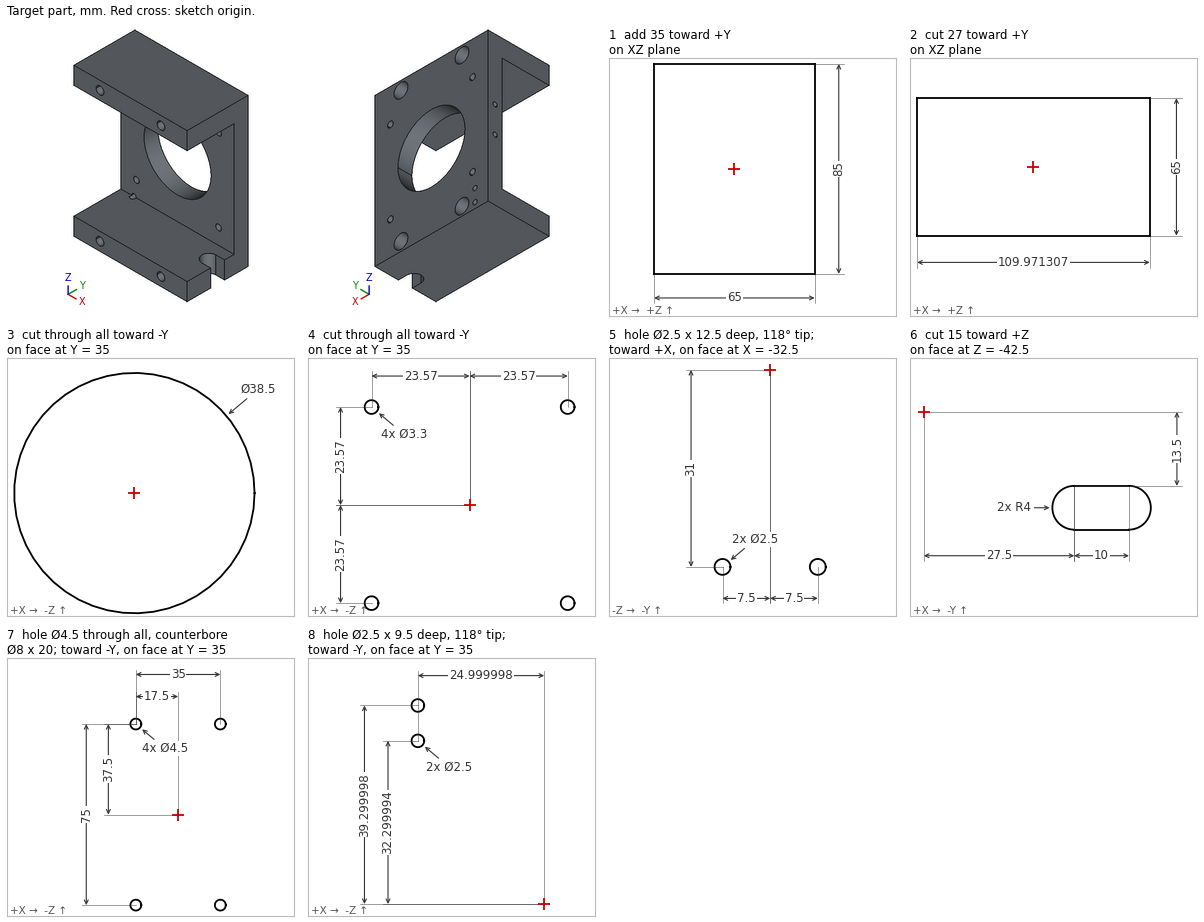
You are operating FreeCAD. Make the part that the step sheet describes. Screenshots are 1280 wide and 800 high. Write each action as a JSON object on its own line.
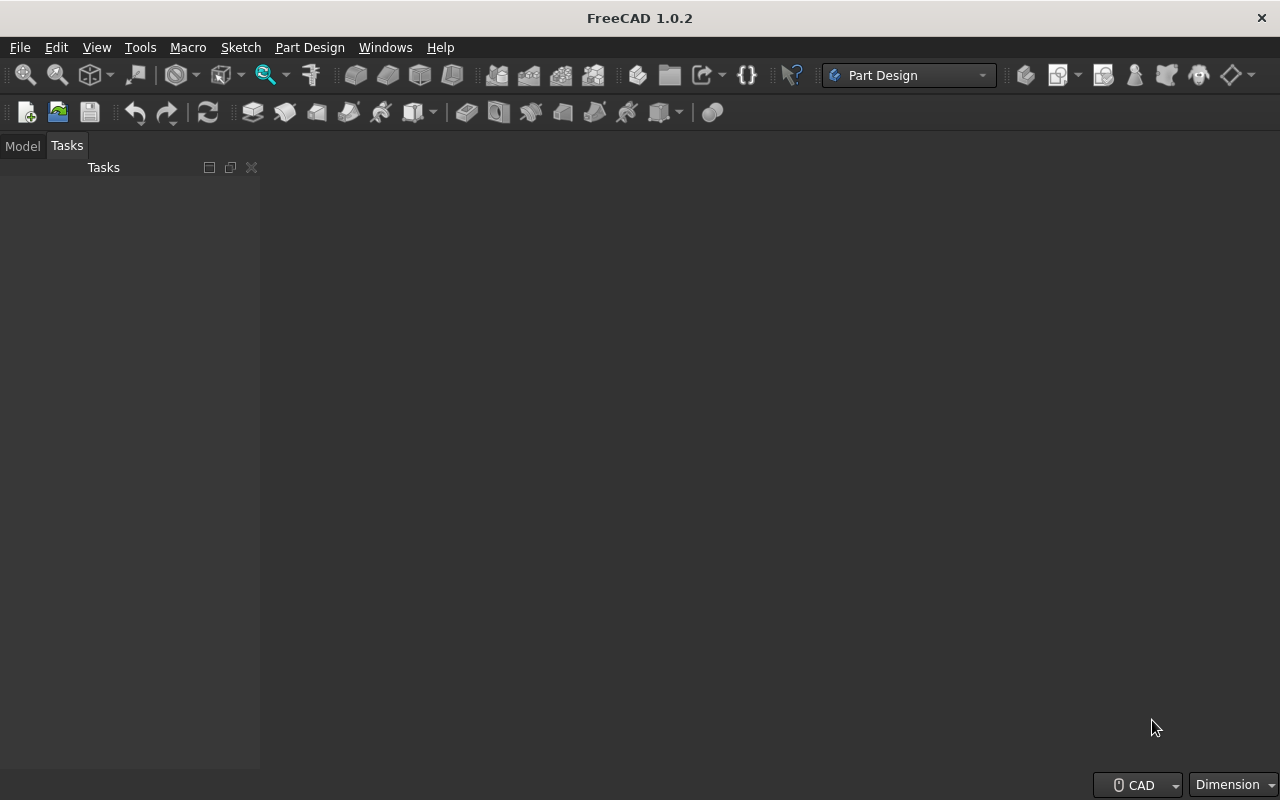
{"action": "left_click", "coordinate": [26, 112]}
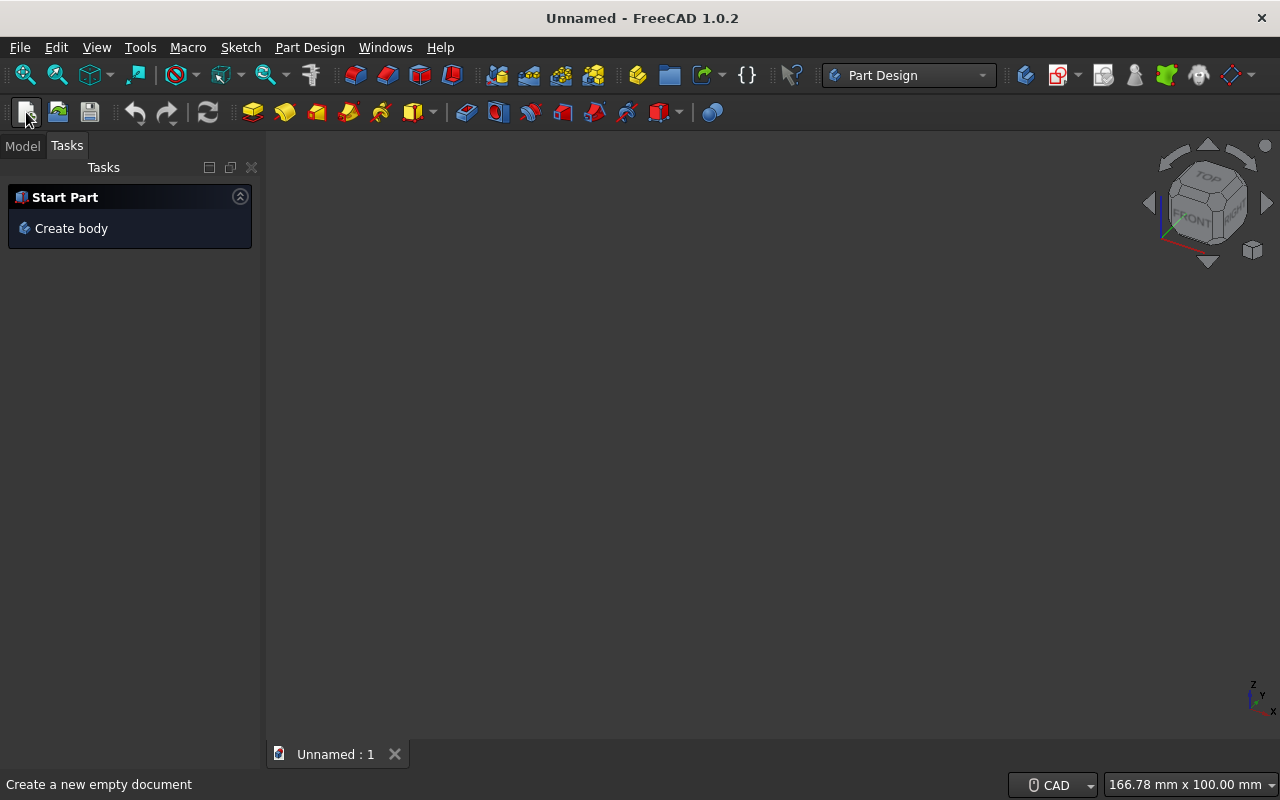
{"action": "left_click", "coordinate": [1058, 76]}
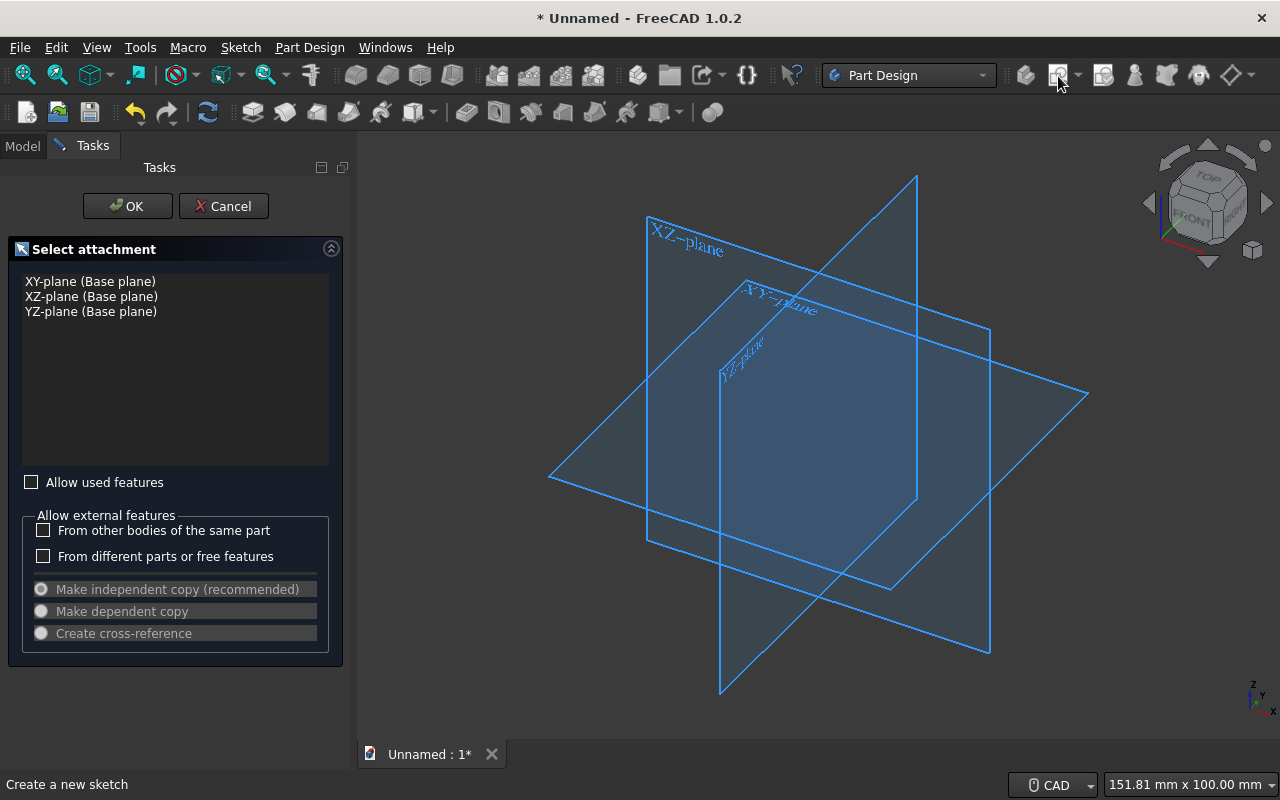
{"action": "left_click", "coordinate": [82, 296]}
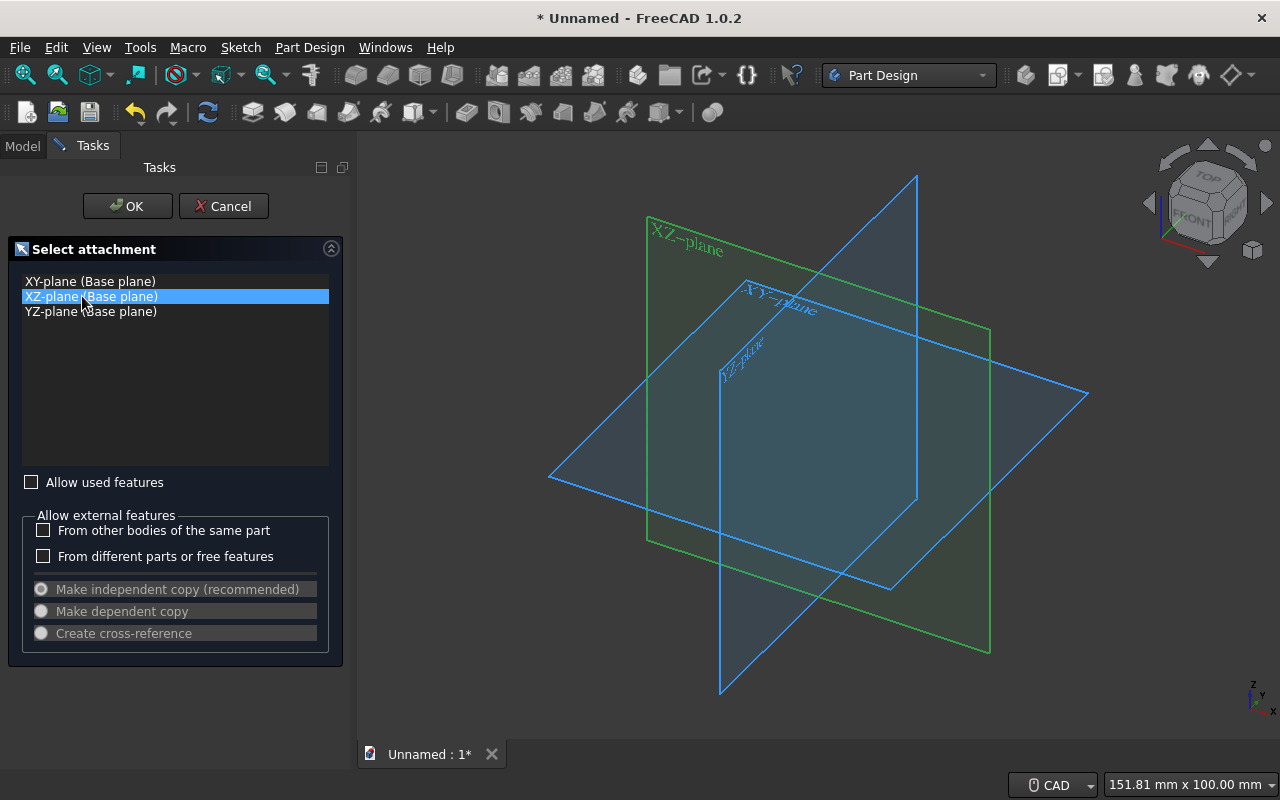
{"action": "left_click", "coordinate": [128, 206]}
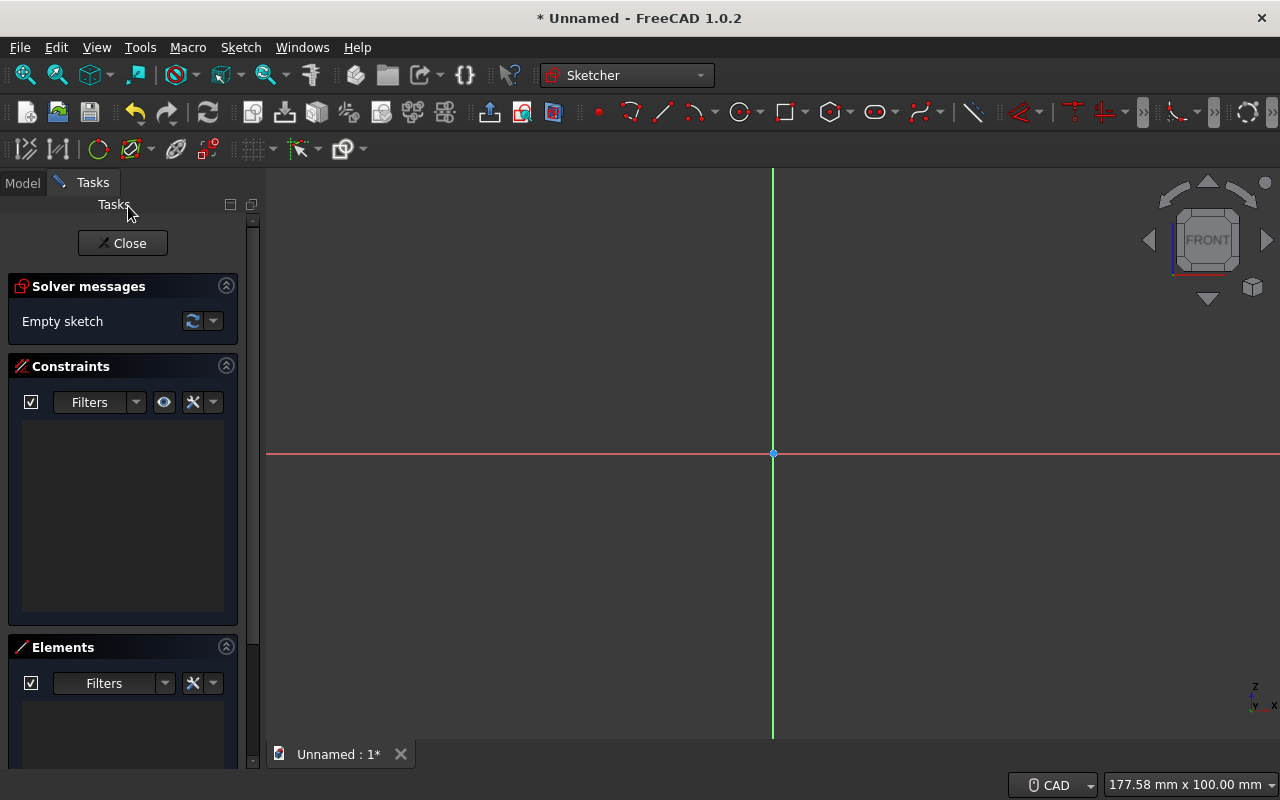
{"action": "scroll", "coordinate": [395, 453], "scroll_direction": "down", "scroll_amount": 1}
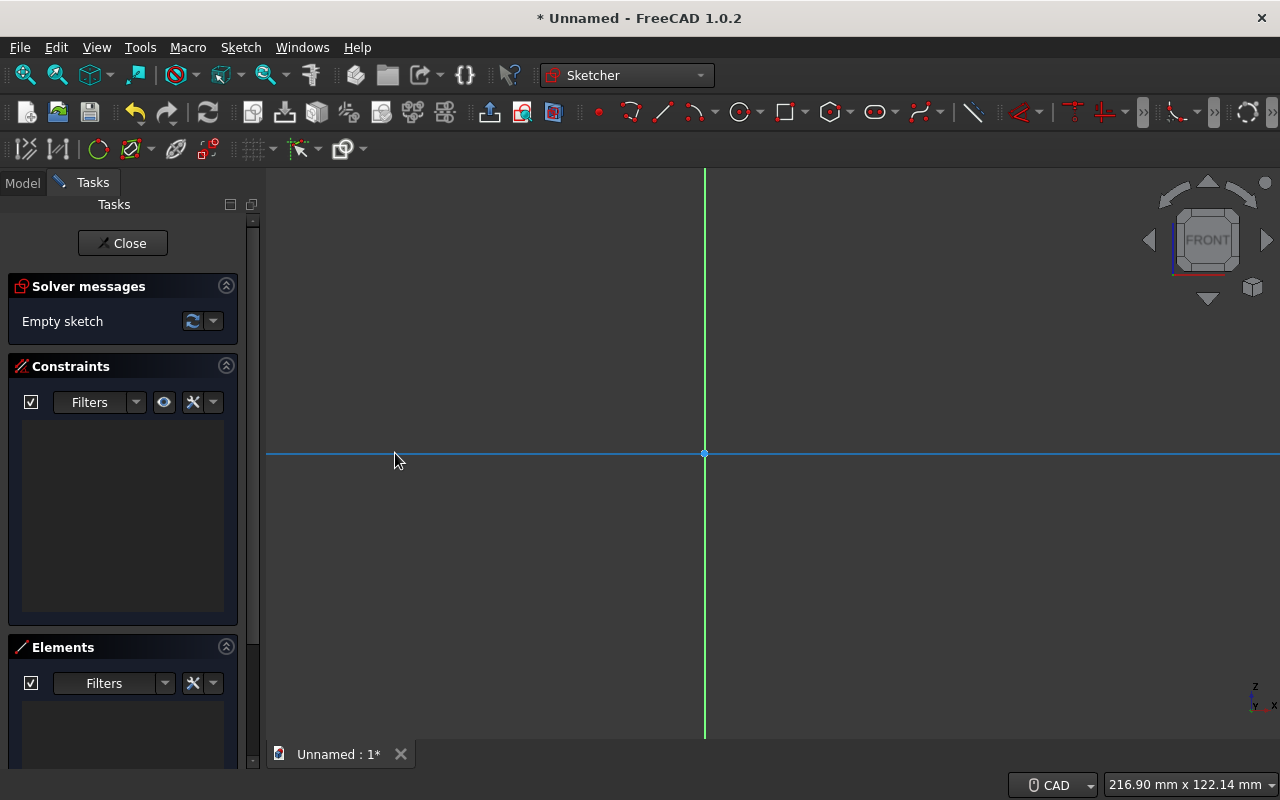
{"action": "left_click", "coordinate": [808, 112]}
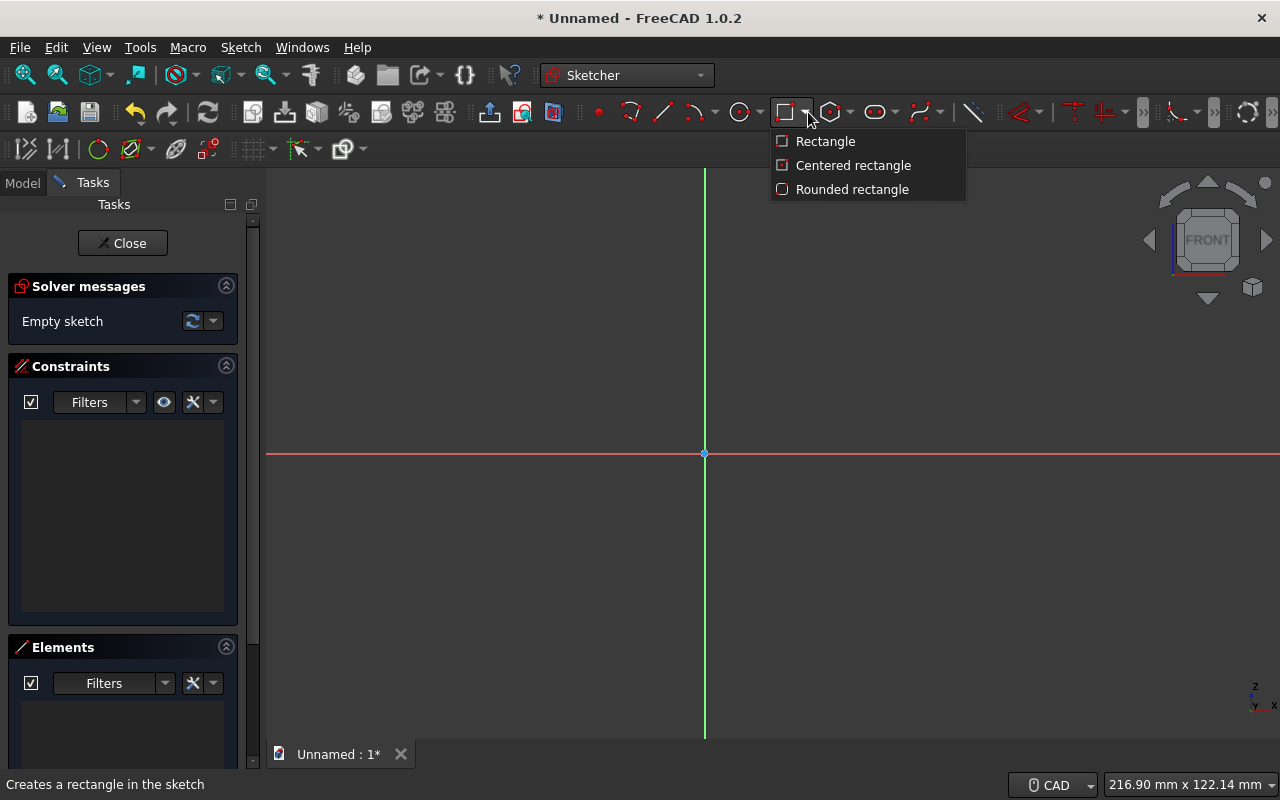
{"action": "left_click", "coordinate": [868, 165]}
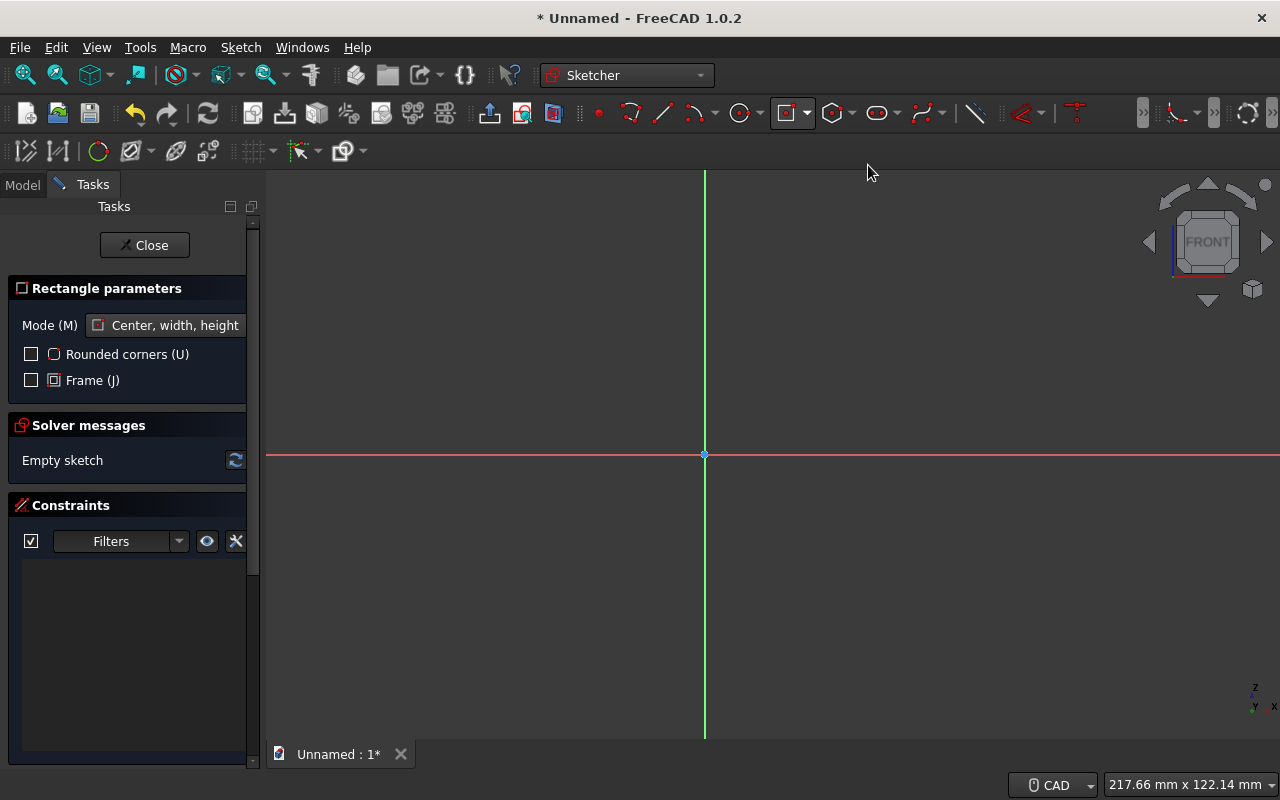
{"action": "left_click", "coordinate": [705, 454]}
{"action": "mouse_move", "coordinate": [856, 257]}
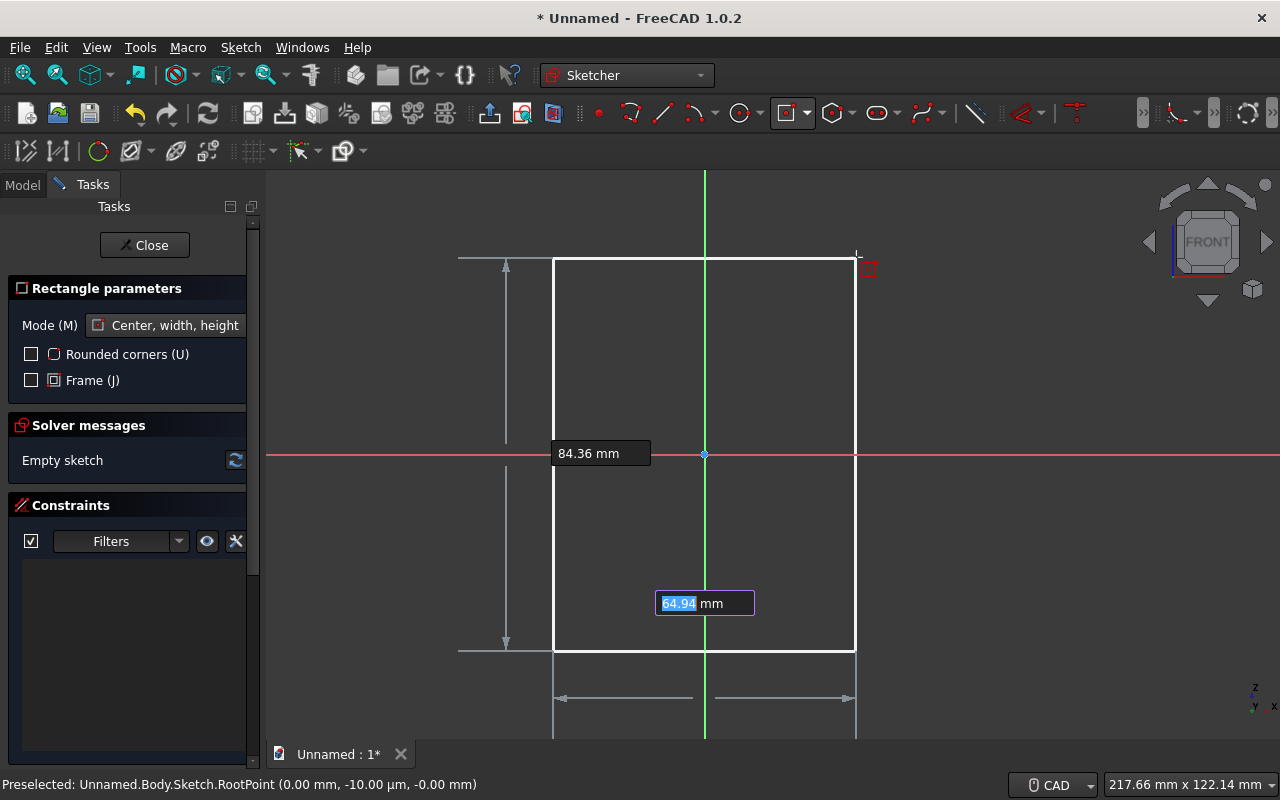
{"action": "type", "text": "65"}
{"action": "key", "text": "Tab"}
{"action": "type", "text": "85"}
{"action": "key", "text": "Return"}
{"action": "key", "text": "Escape"}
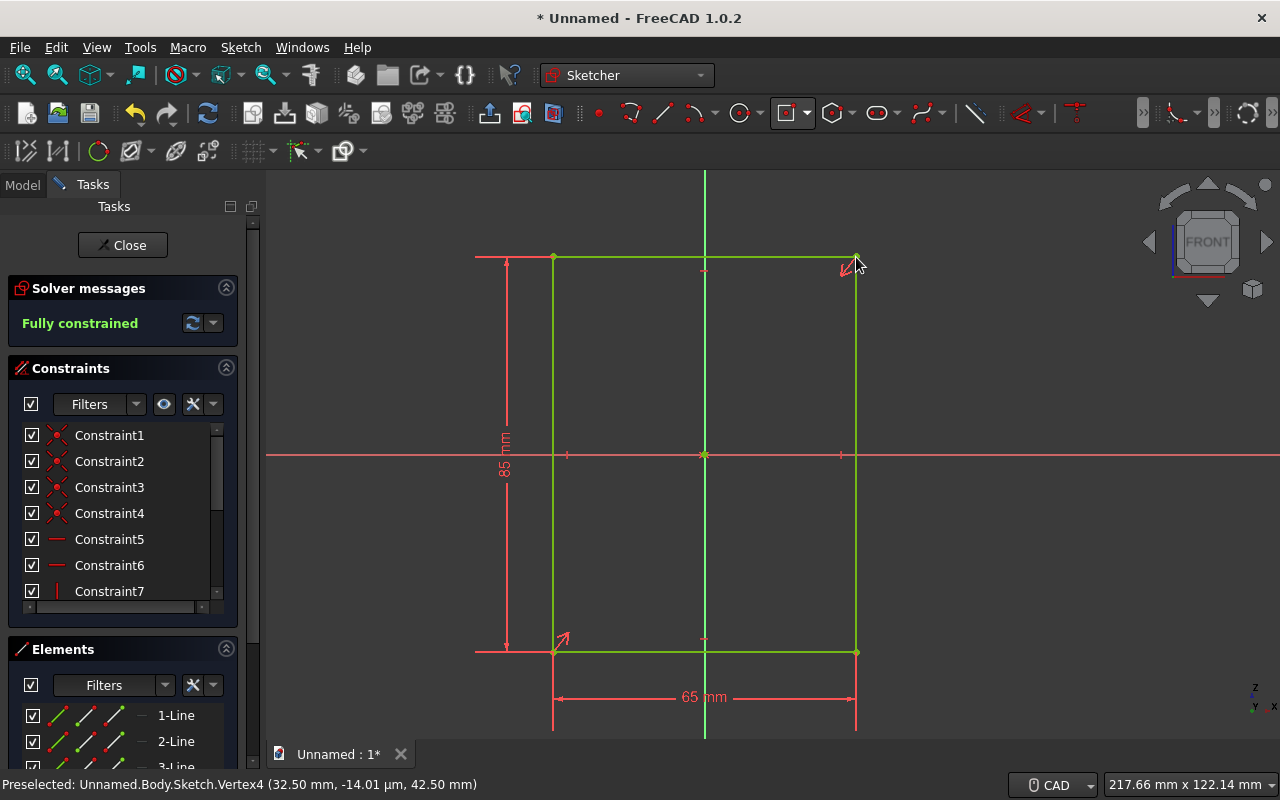
{"action": "left_click", "coordinate": [123, 245]}